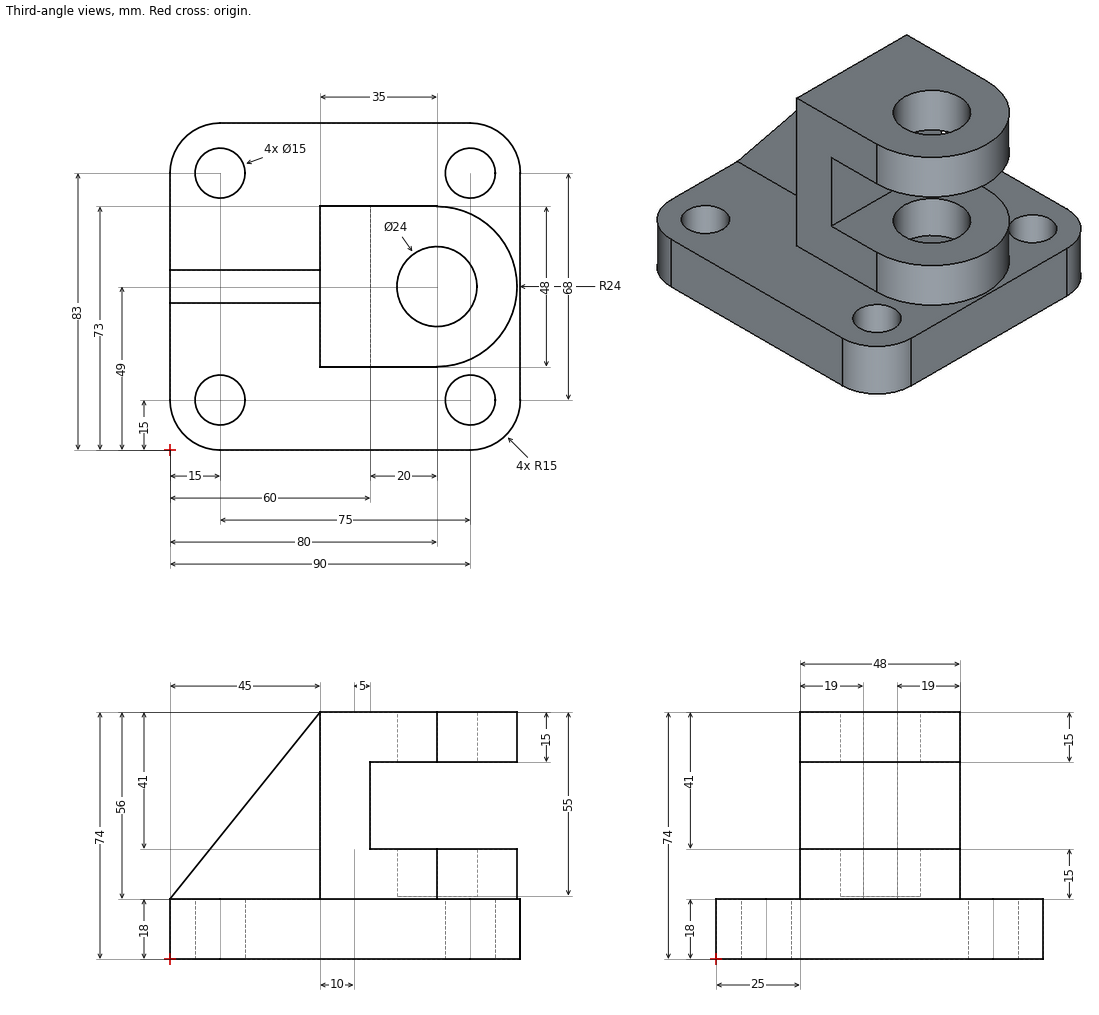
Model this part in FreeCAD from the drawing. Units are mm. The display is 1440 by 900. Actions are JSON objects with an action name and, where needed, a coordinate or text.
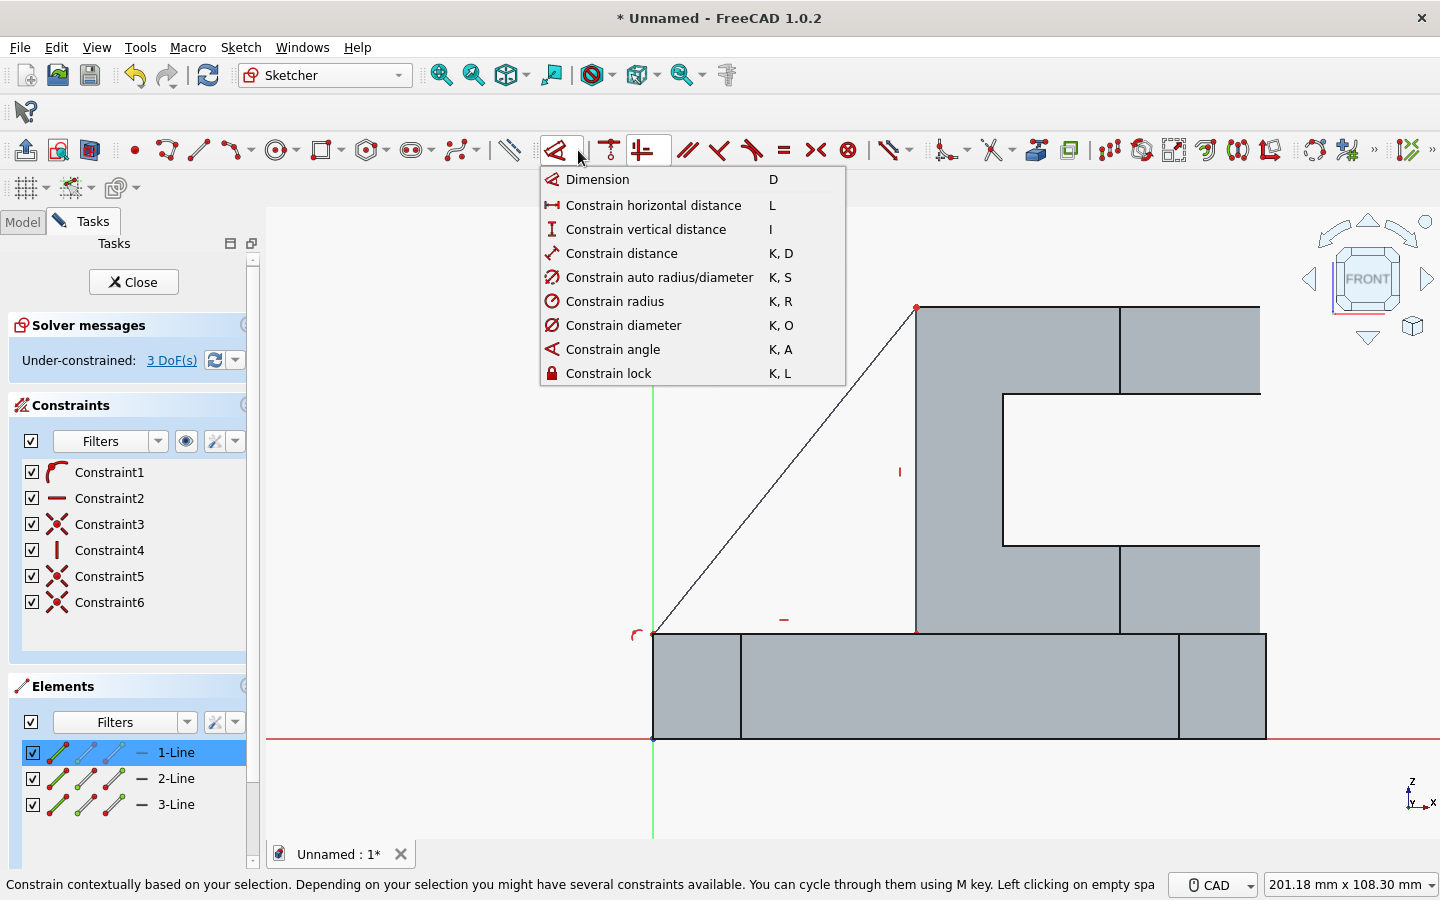
{"action": "left_click", "coordinate": [693, 205]}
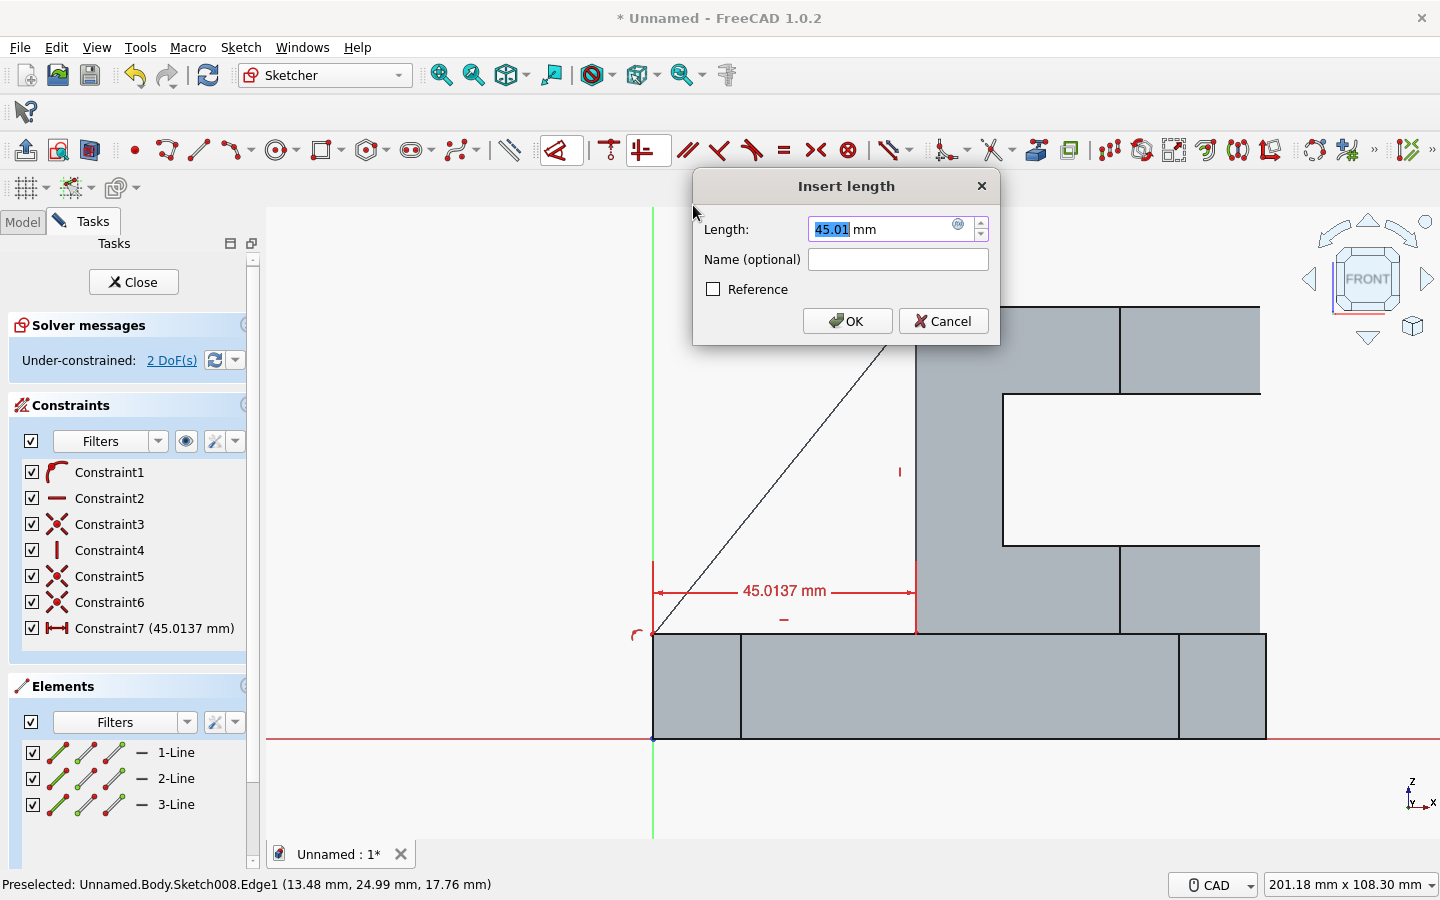
{"action": "type", "text": "45"}
{"action": "key", "text": "Return"}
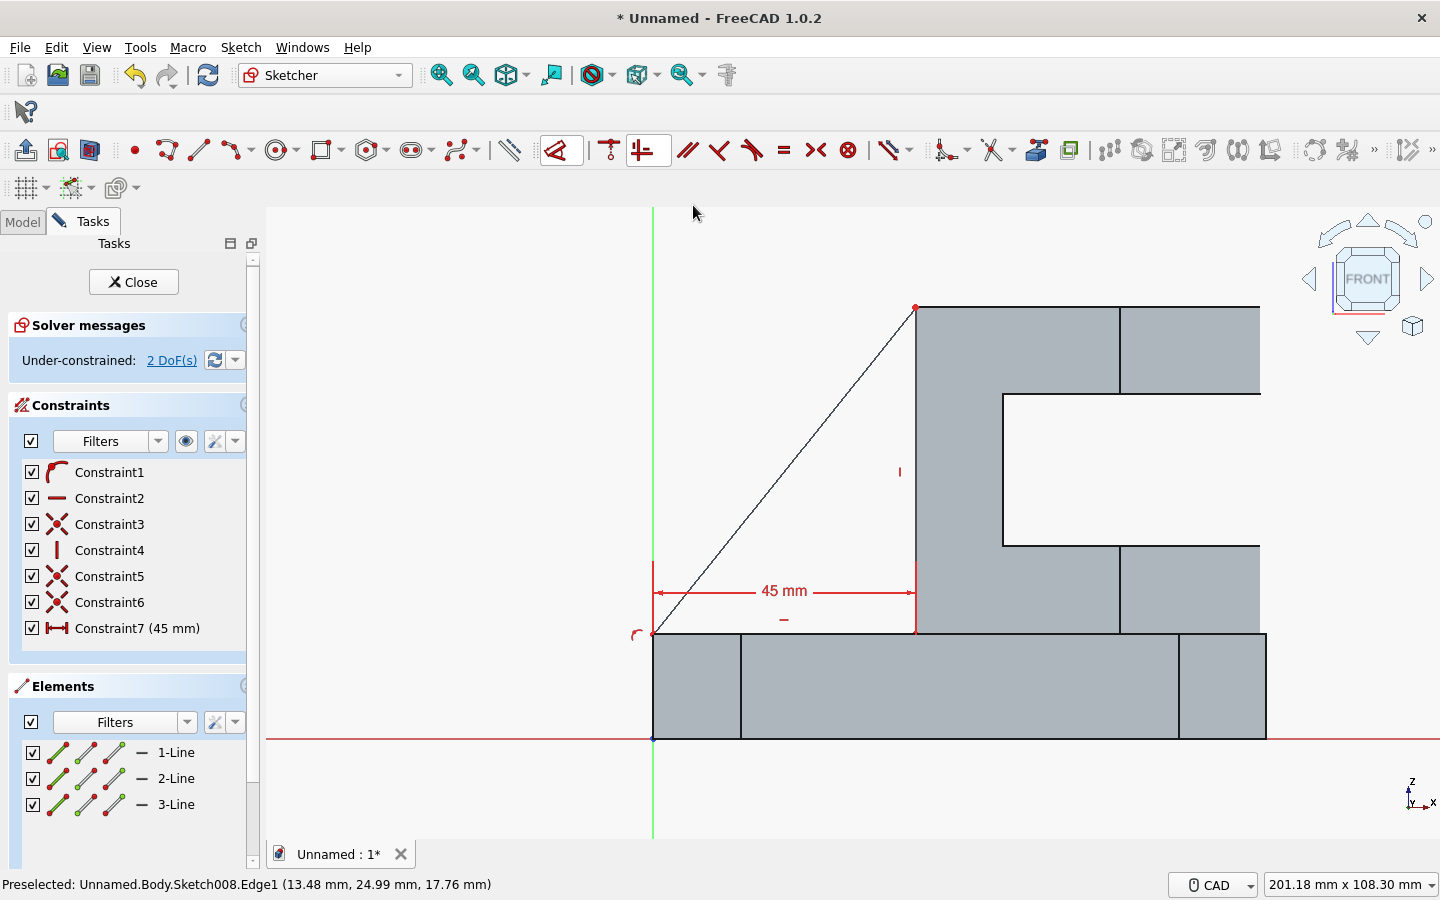
{"action": "left_click", "coordinate": [916, 537]}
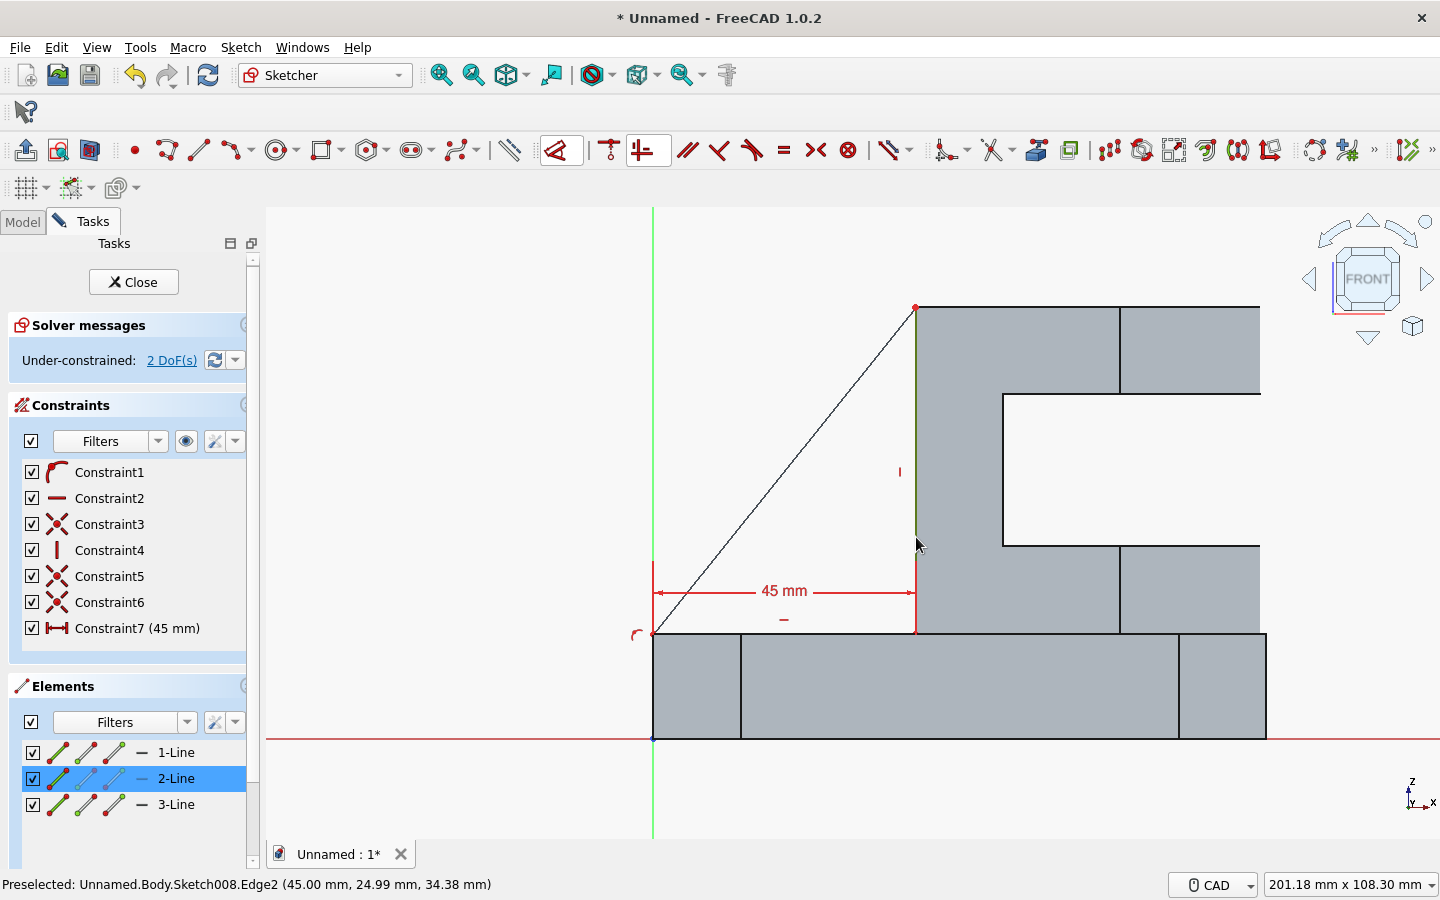
{"action": "key", "text": "i"}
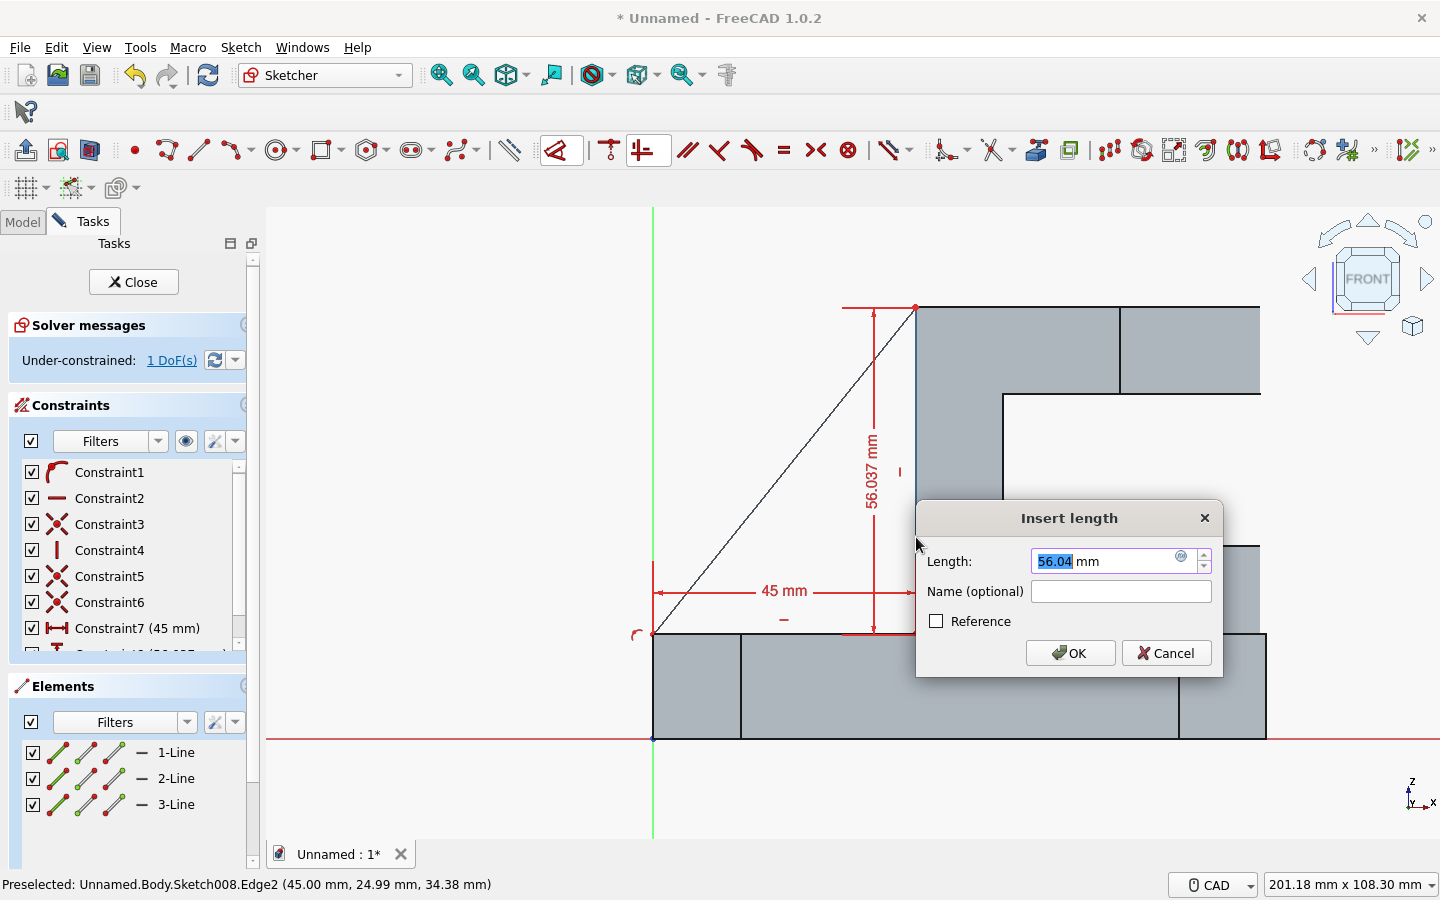
{"action": "type", "text": "56"}
{"action": "key", "text": "Return"}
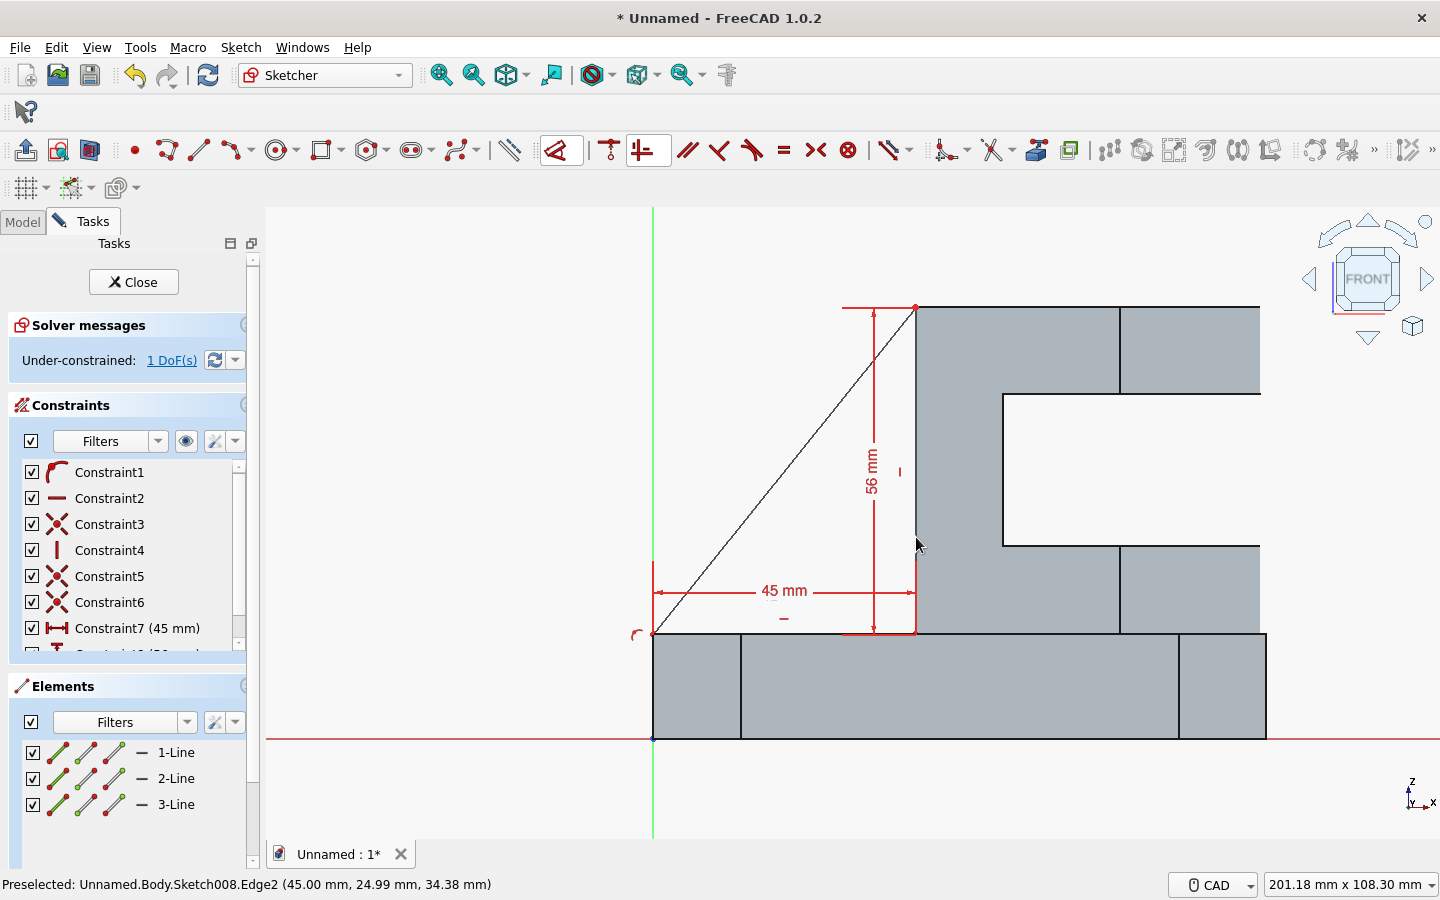
{"action": "left_click", "coordinate": [653, 635]}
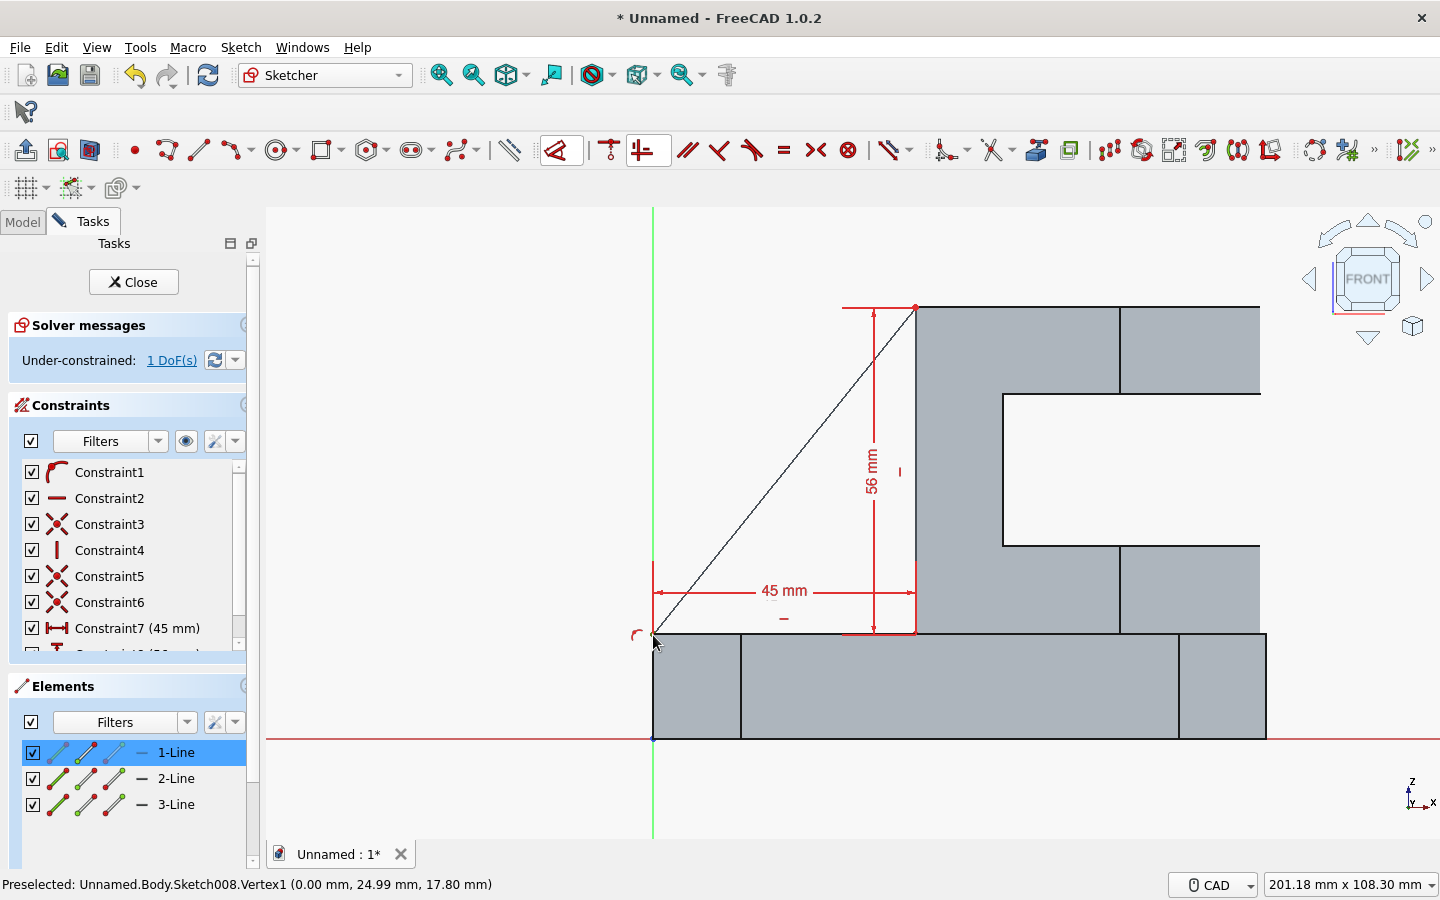
{"action": "left_click", "coordinate": [578, 150]}